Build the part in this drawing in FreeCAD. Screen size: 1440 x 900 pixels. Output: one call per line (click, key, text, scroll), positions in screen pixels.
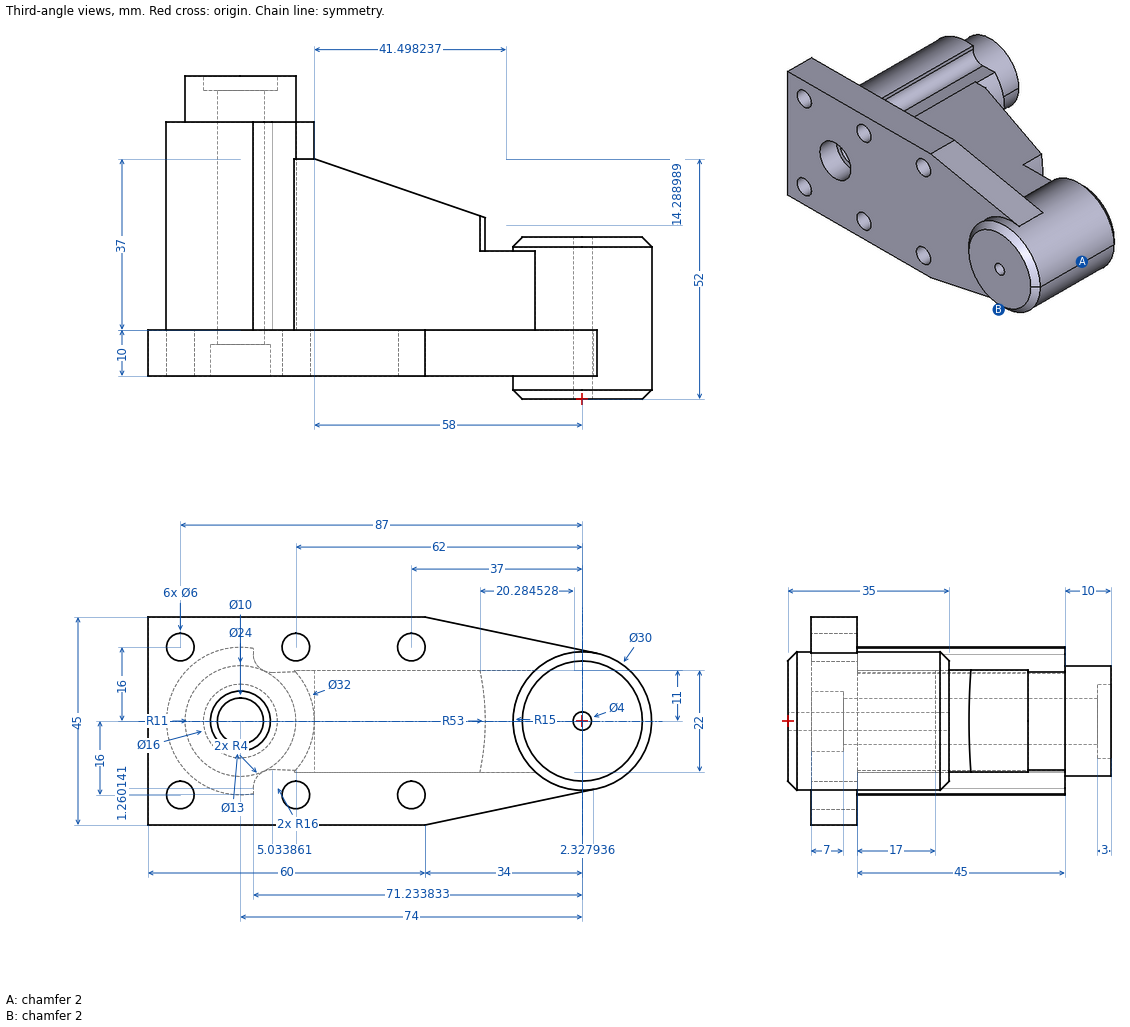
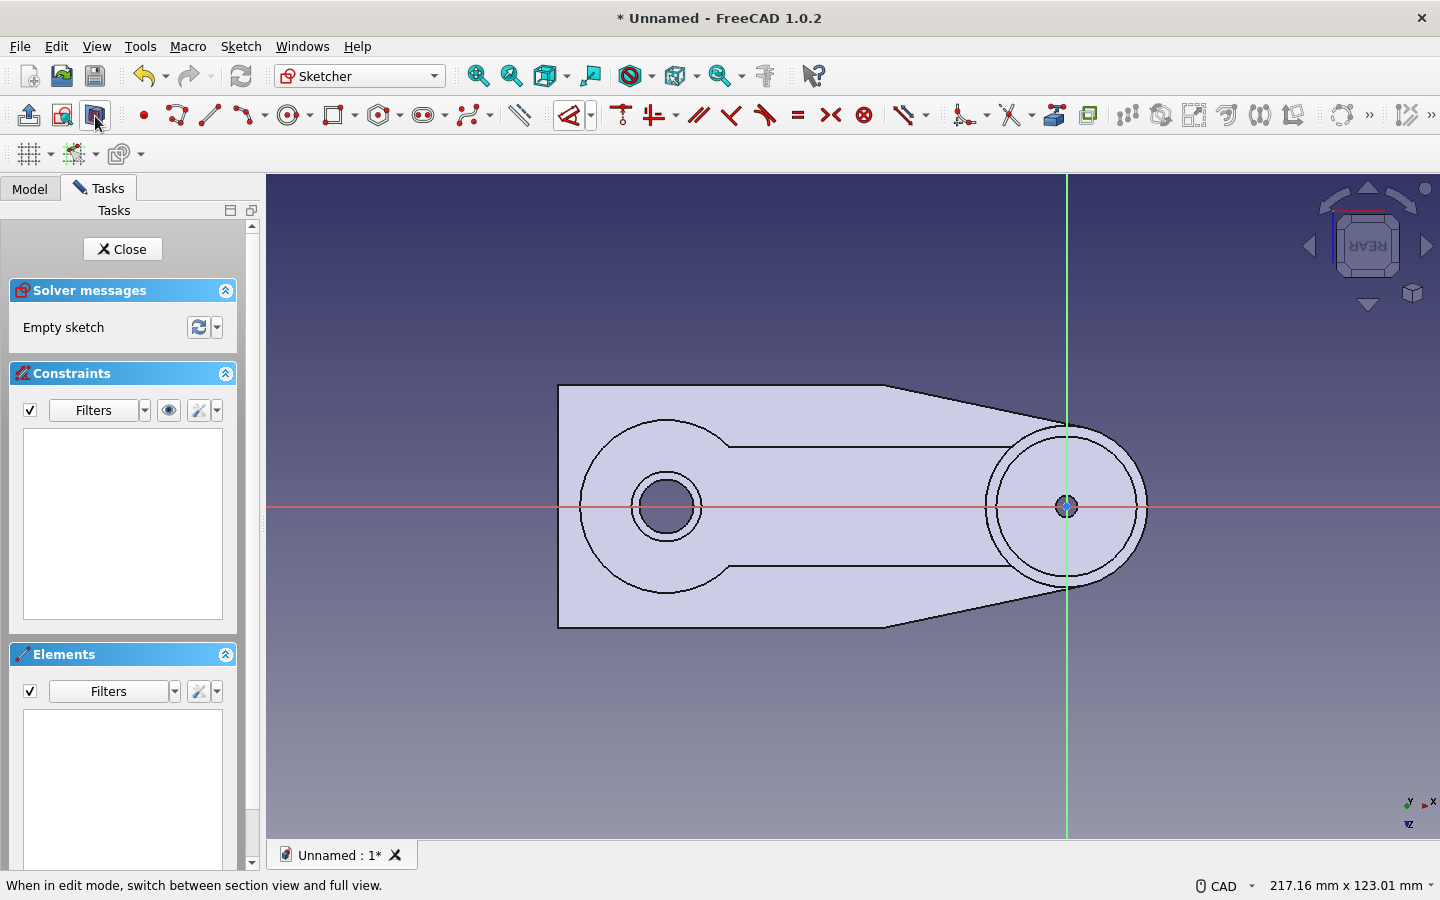
scroll(983, 506, up, 3)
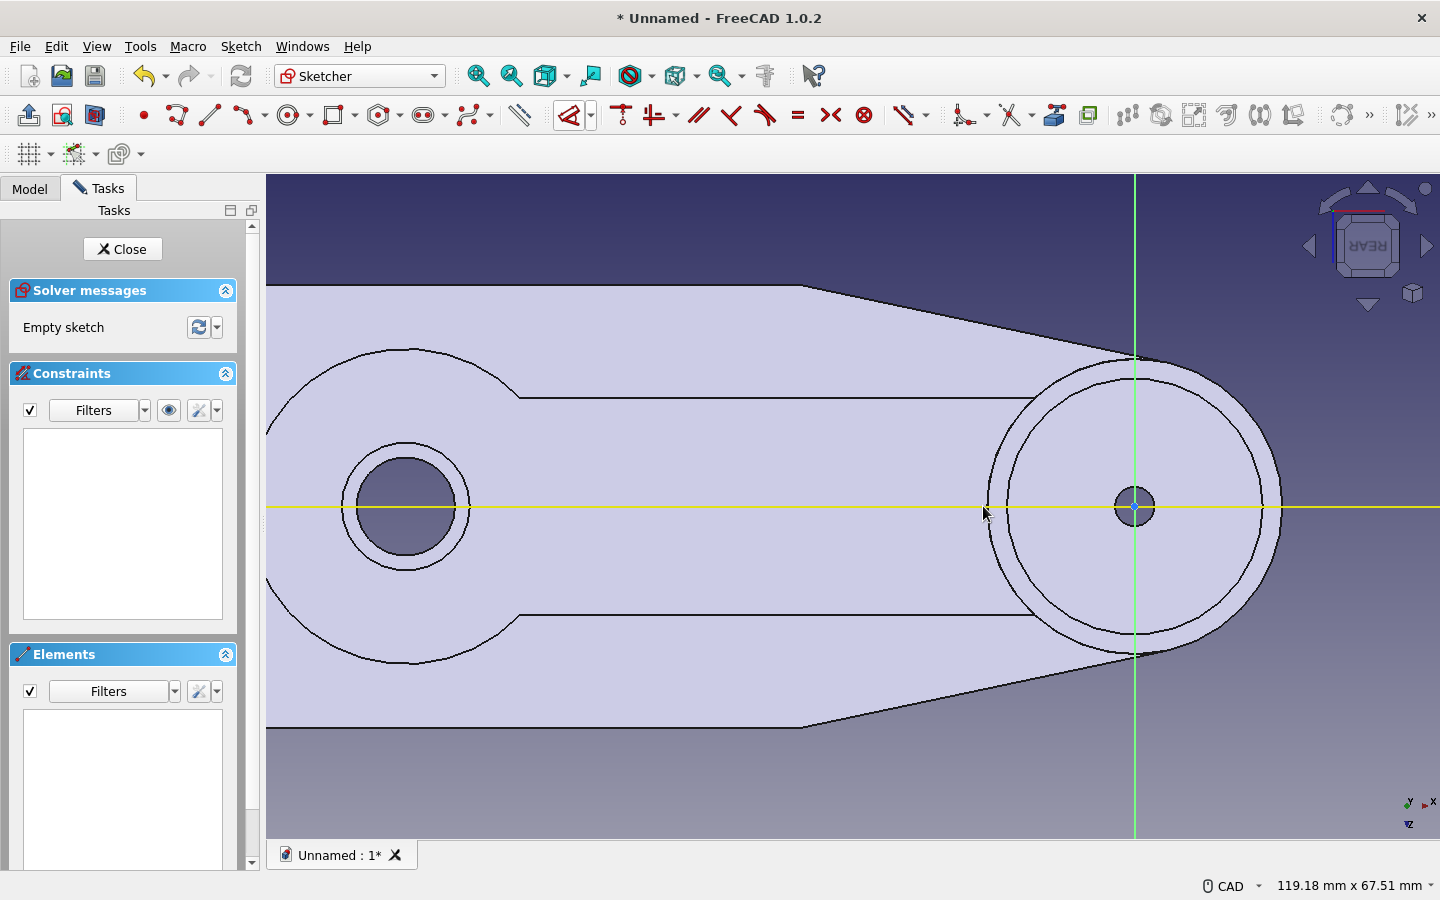
click(210, 116)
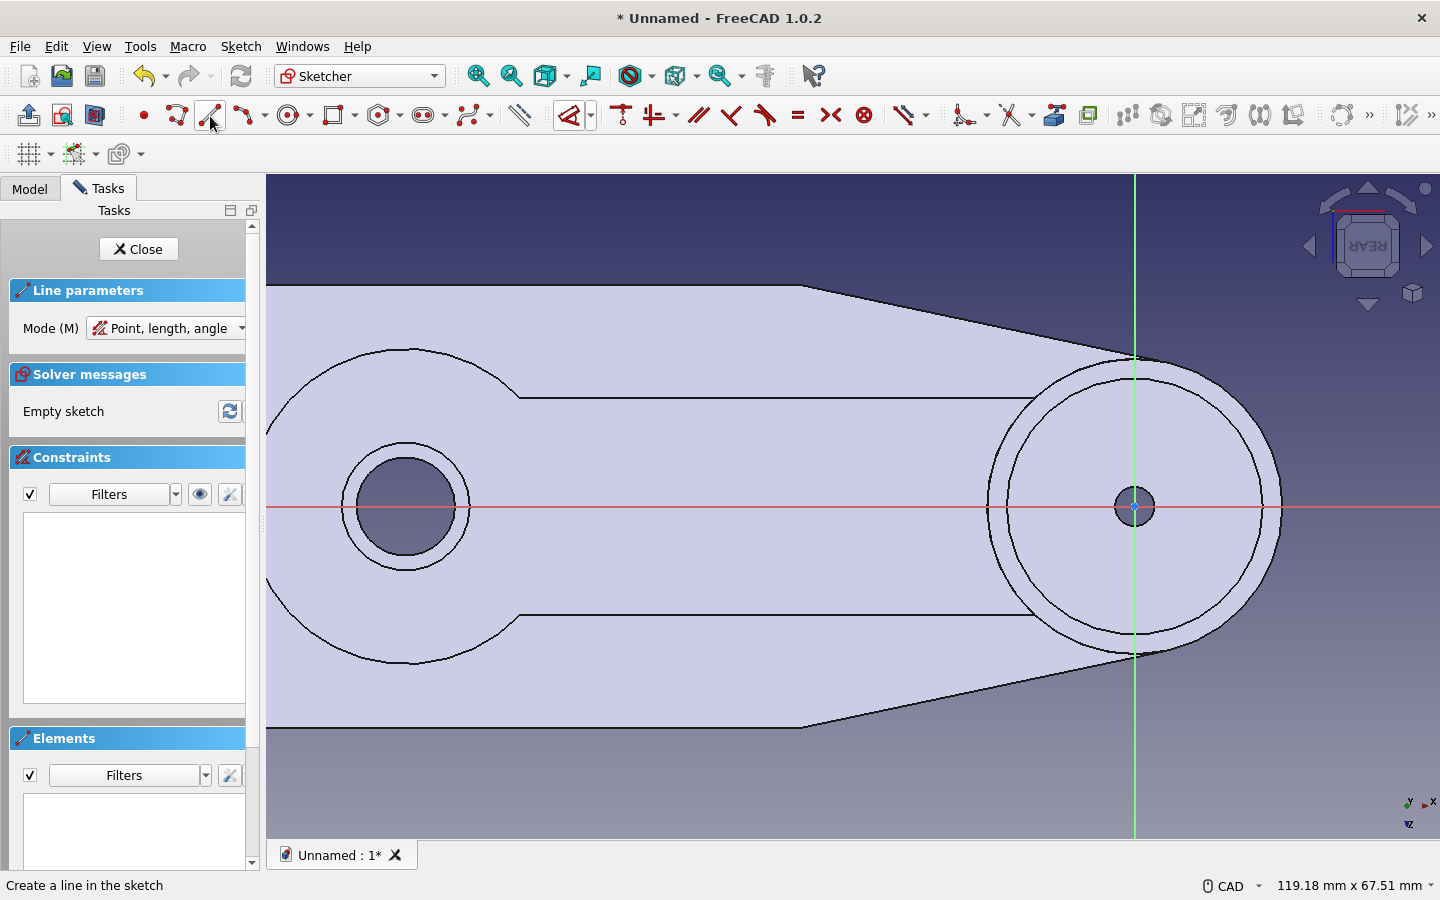
click(433, 351)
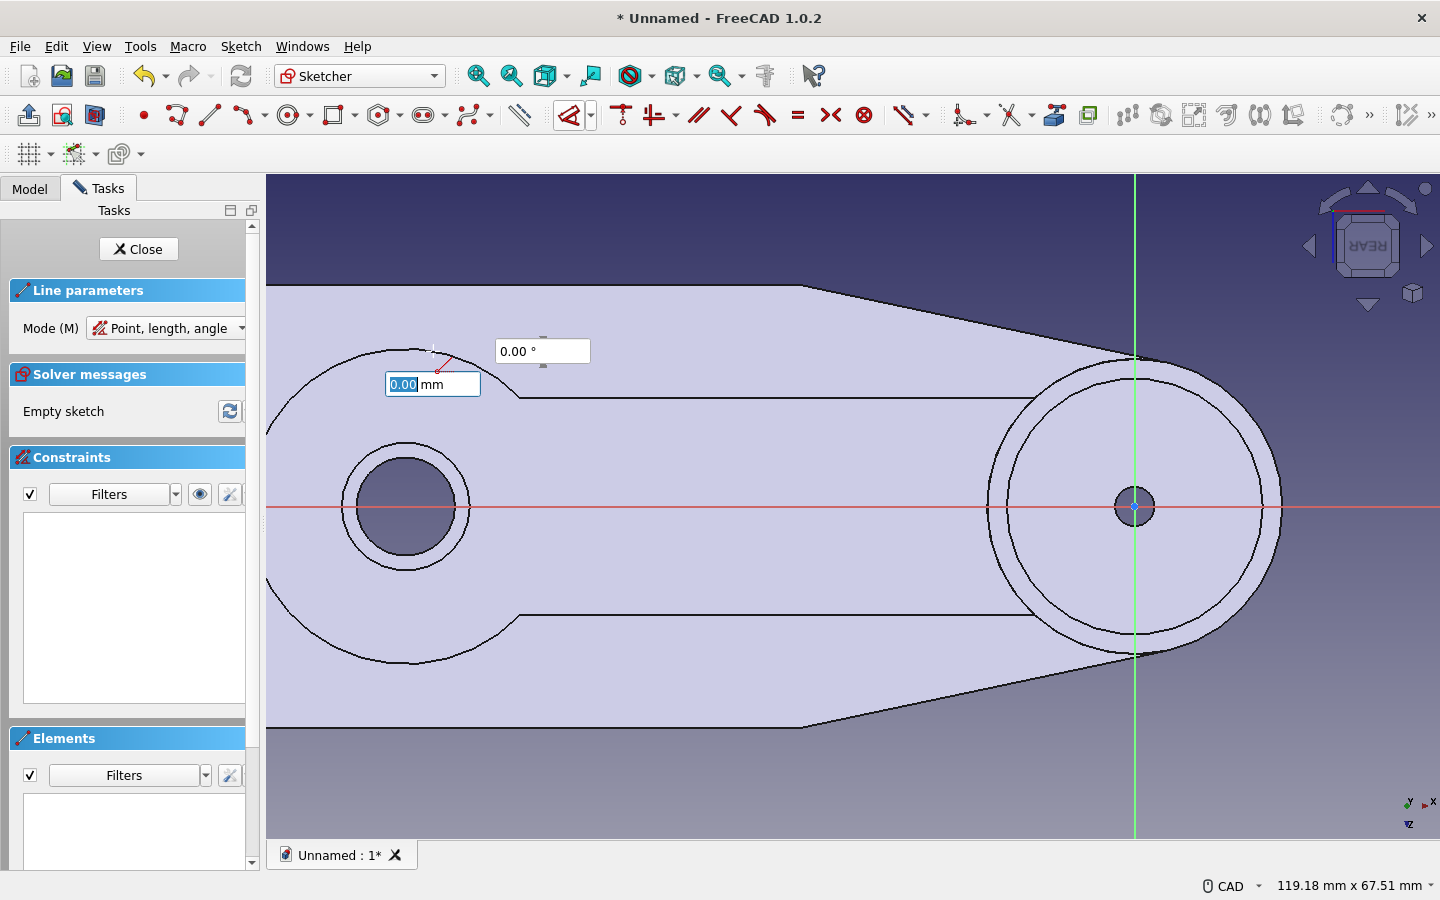
scroll(433, 364, up, 2)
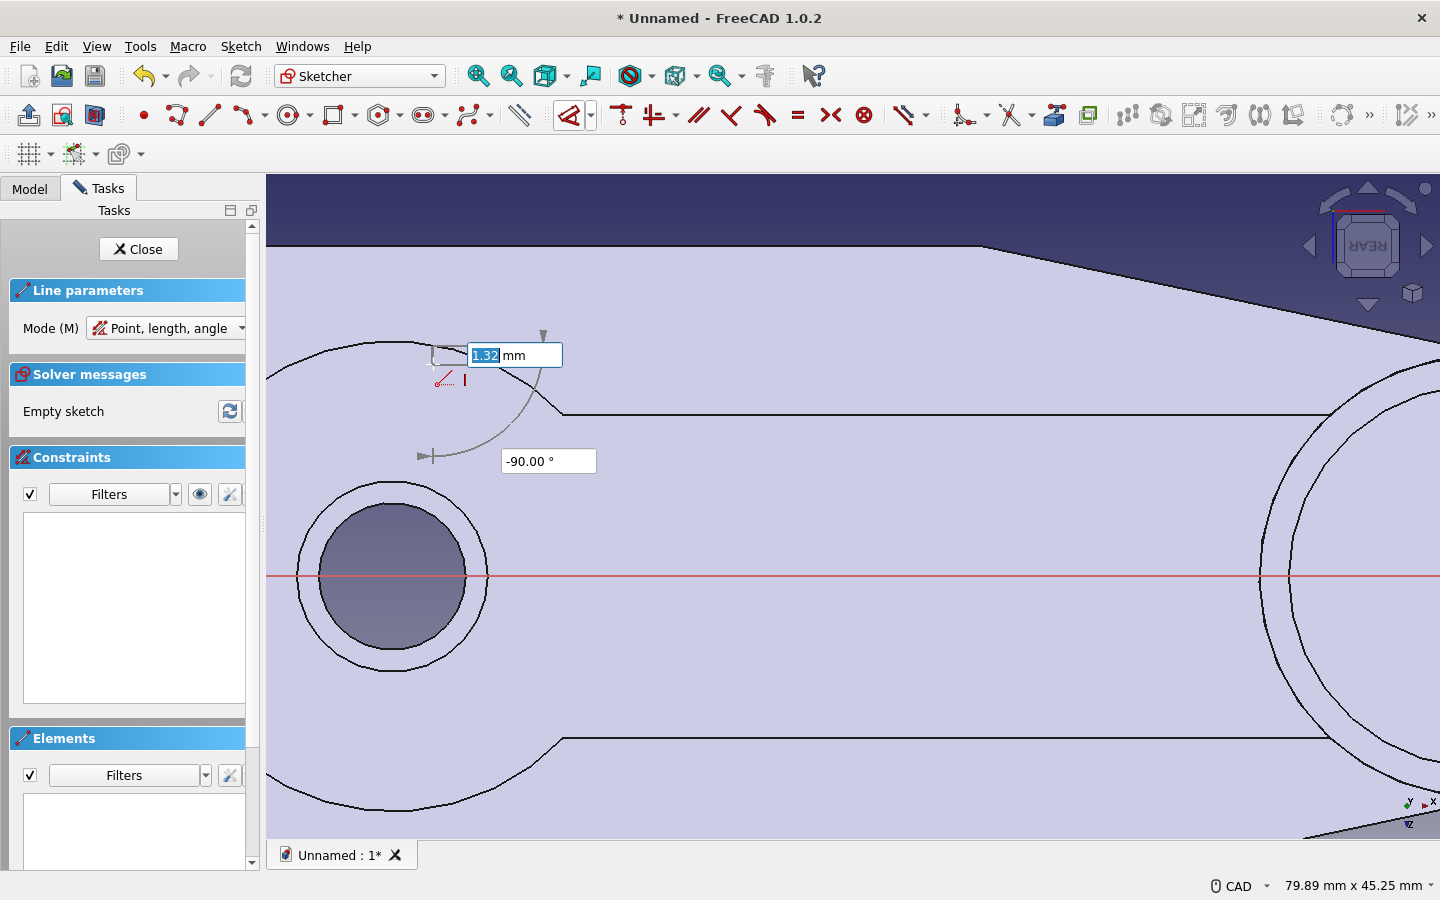
click(433, 363)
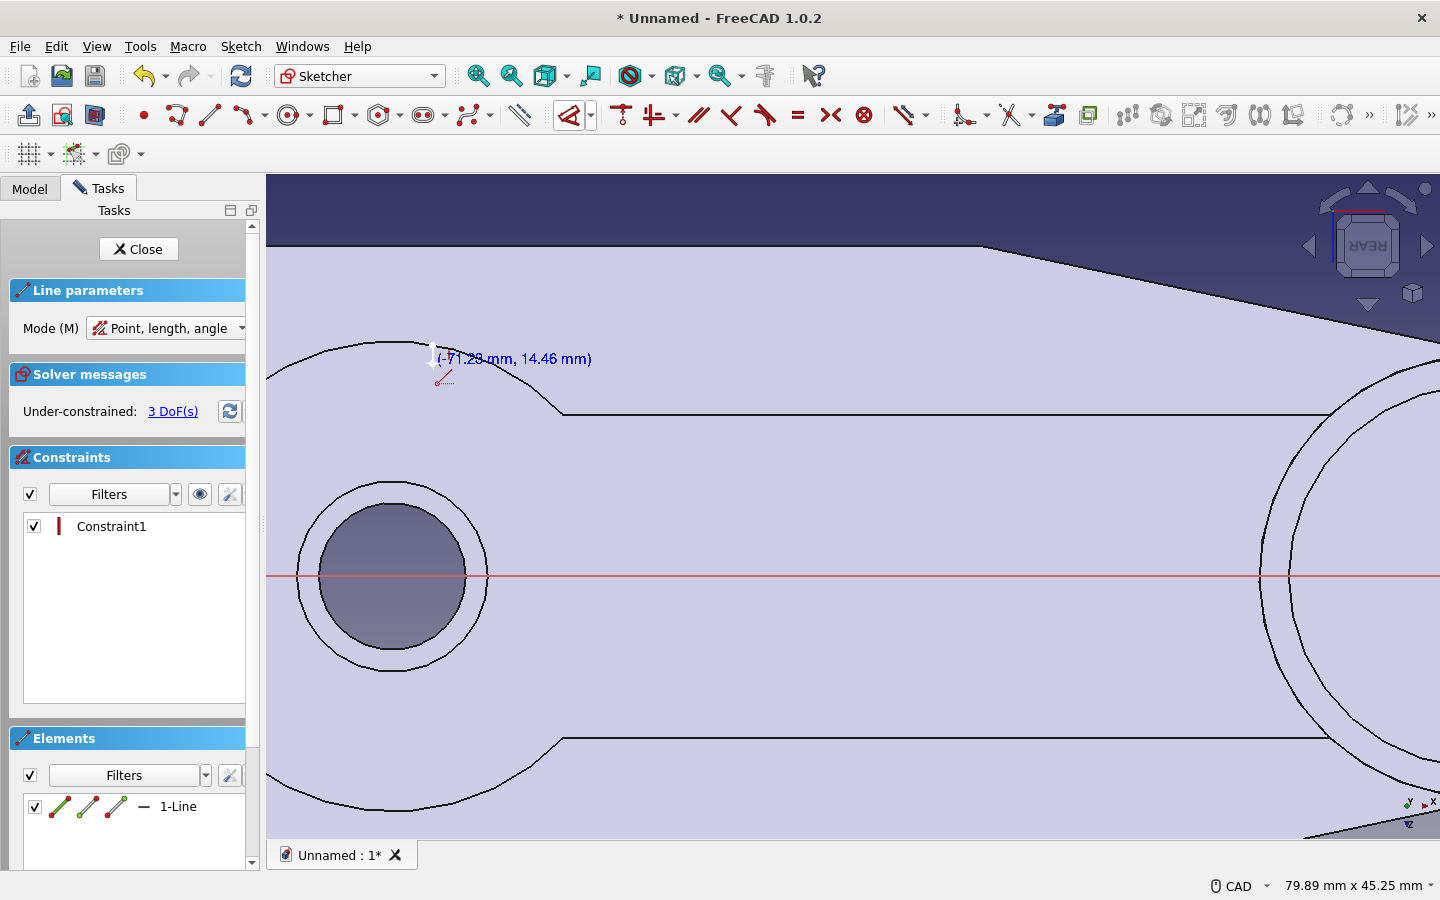
click(494, 422)
click(568, 417)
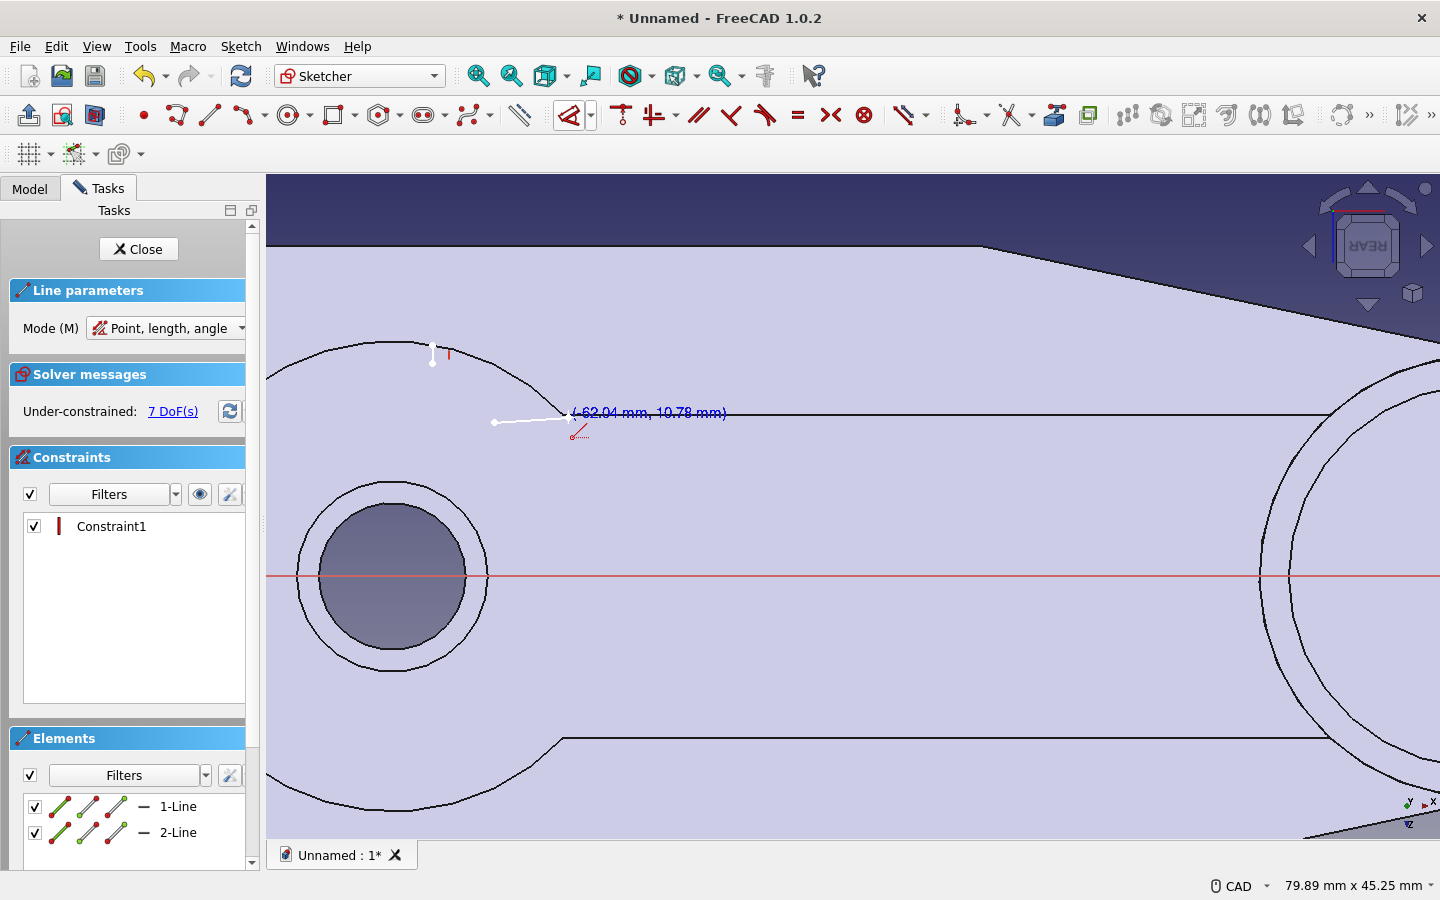
click(242, 116)